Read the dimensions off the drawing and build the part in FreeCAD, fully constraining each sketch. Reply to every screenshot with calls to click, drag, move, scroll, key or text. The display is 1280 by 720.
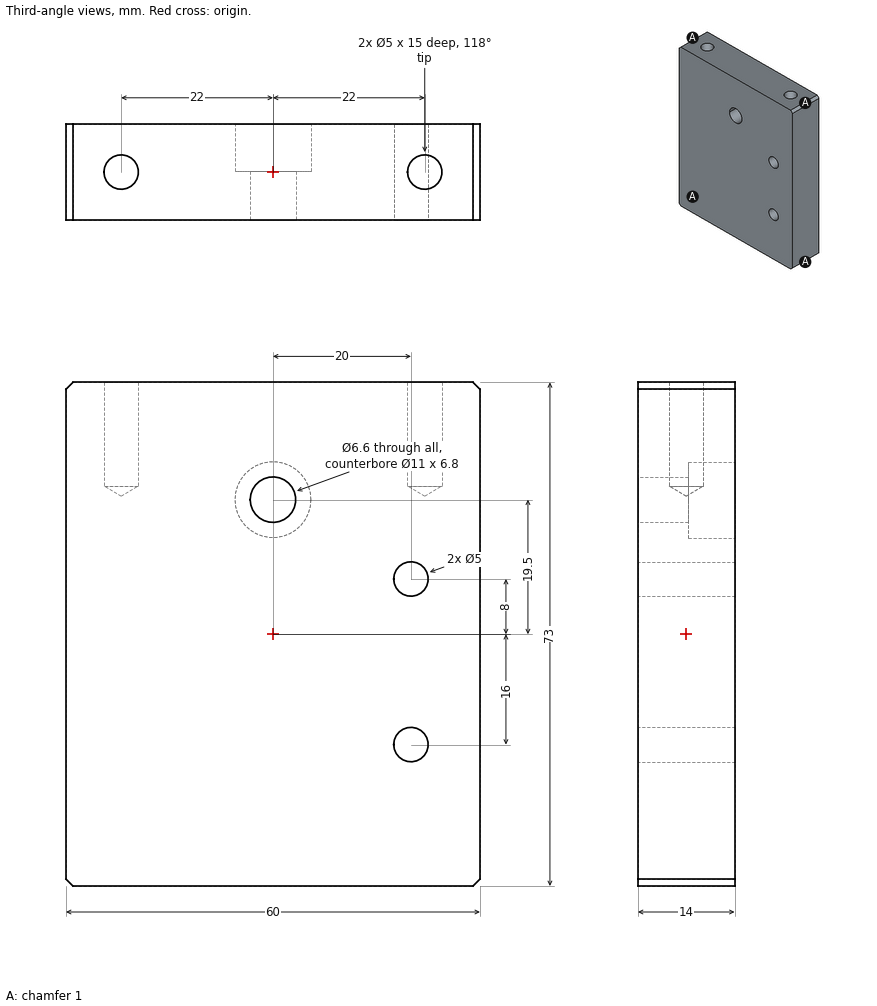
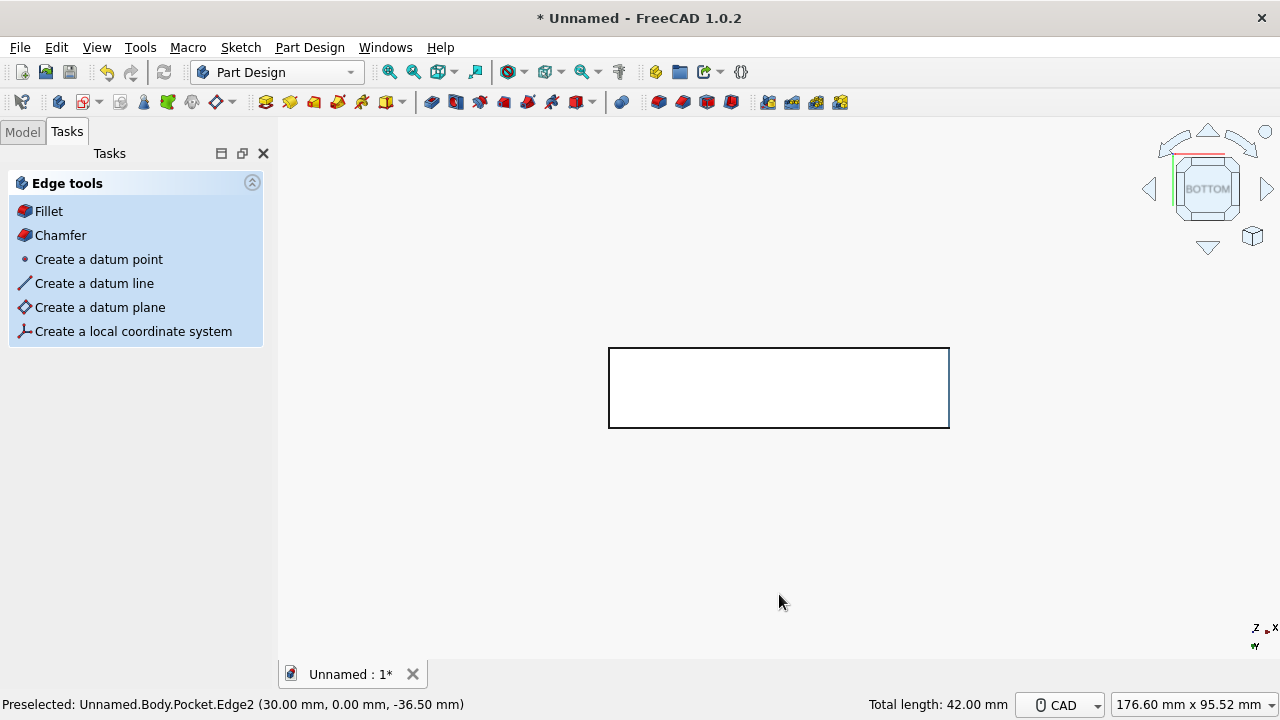
click(390, 72)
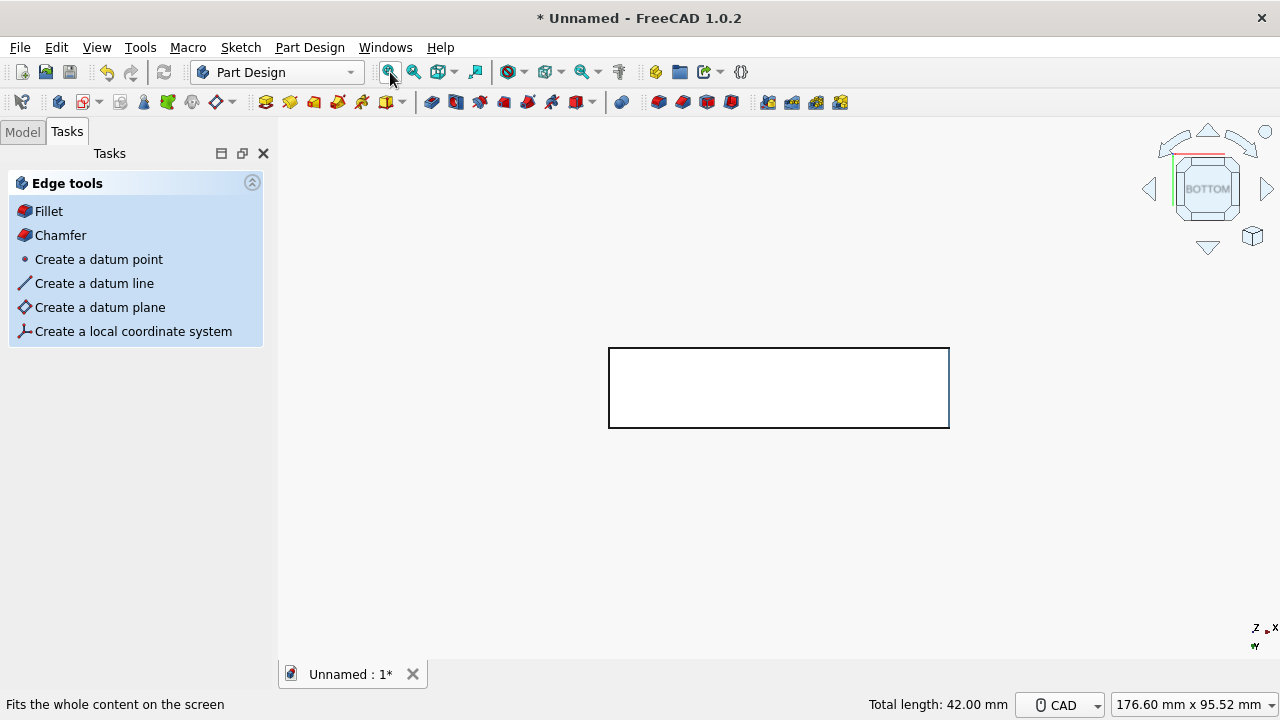
click(609, 387, ctrl)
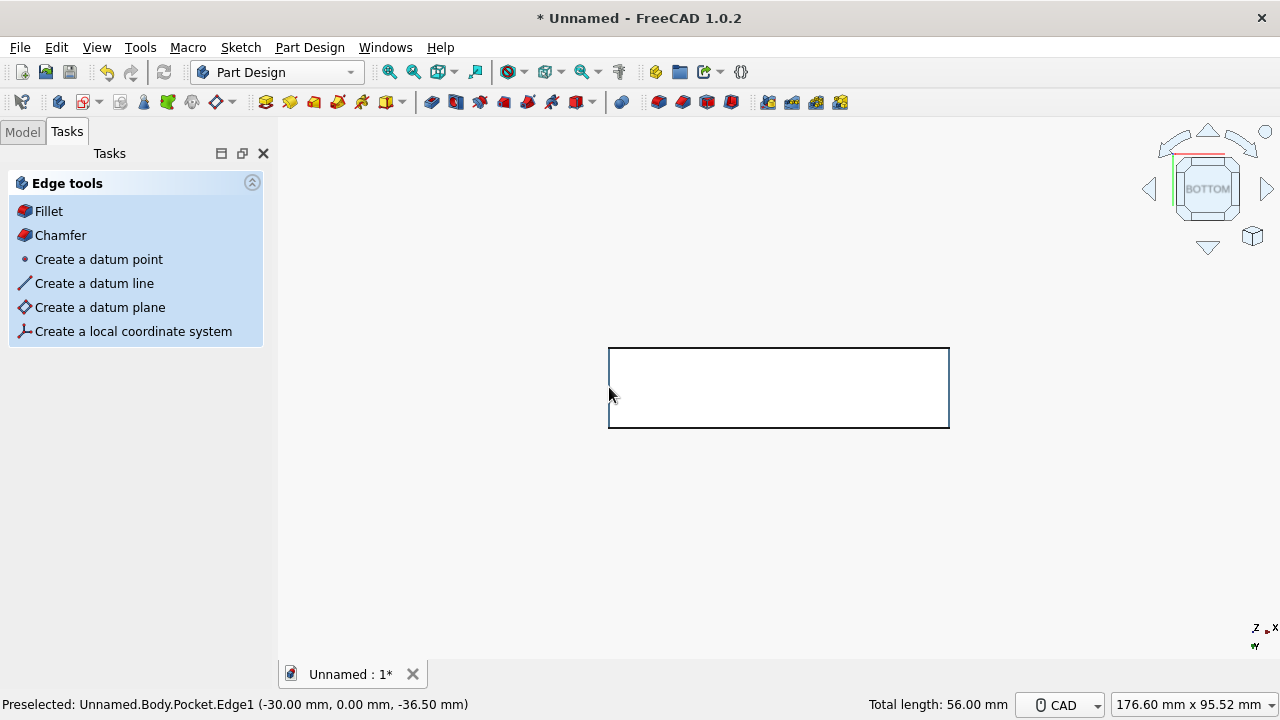
click(684, 102)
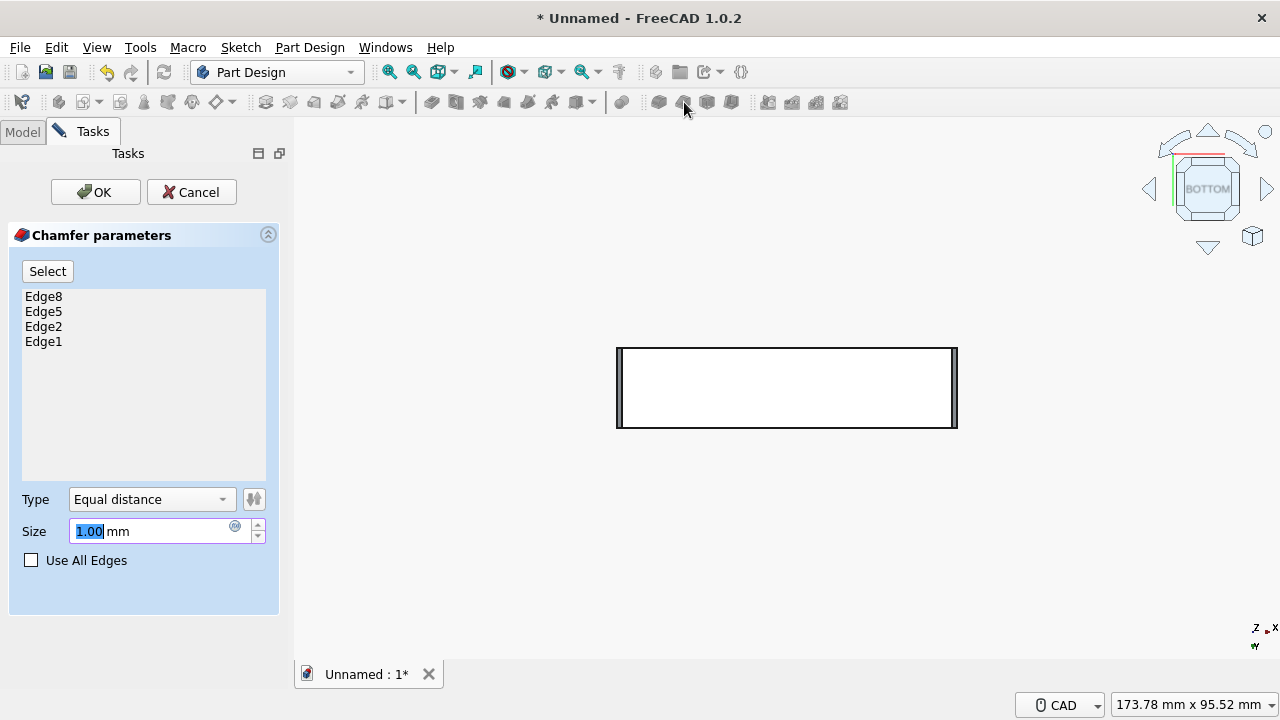
text(1)
key(Tab)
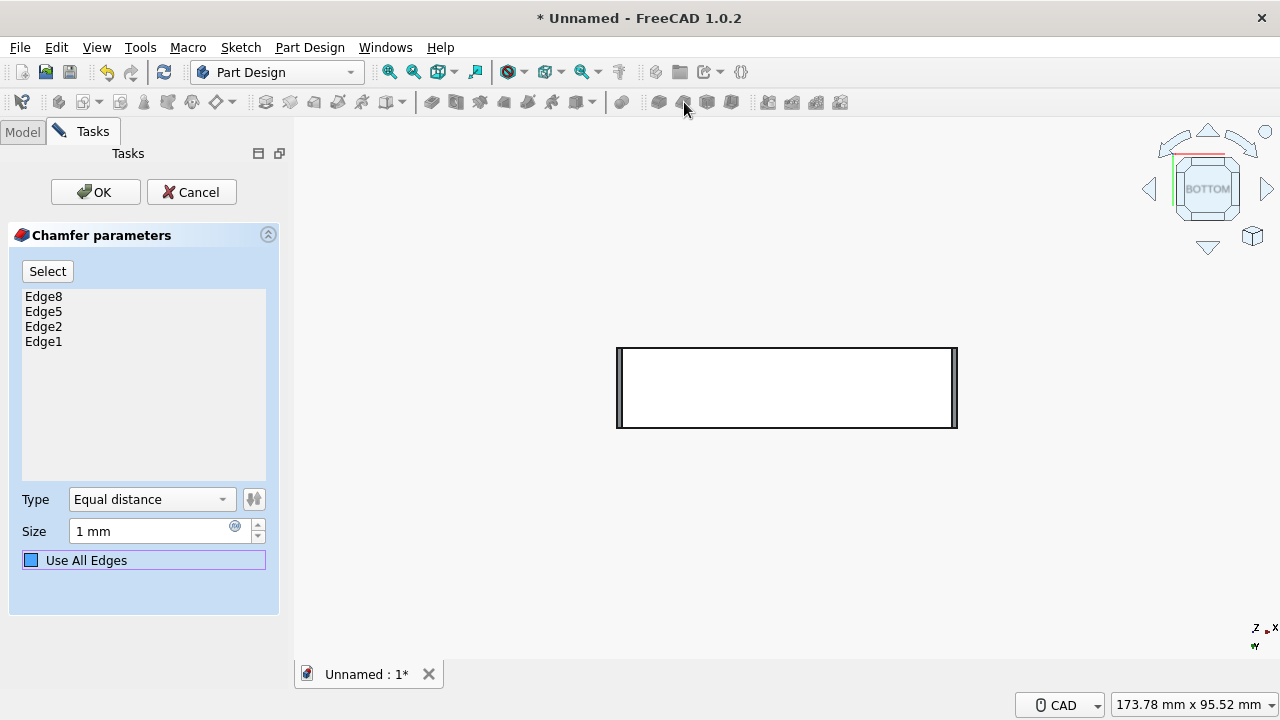
click(96, 192)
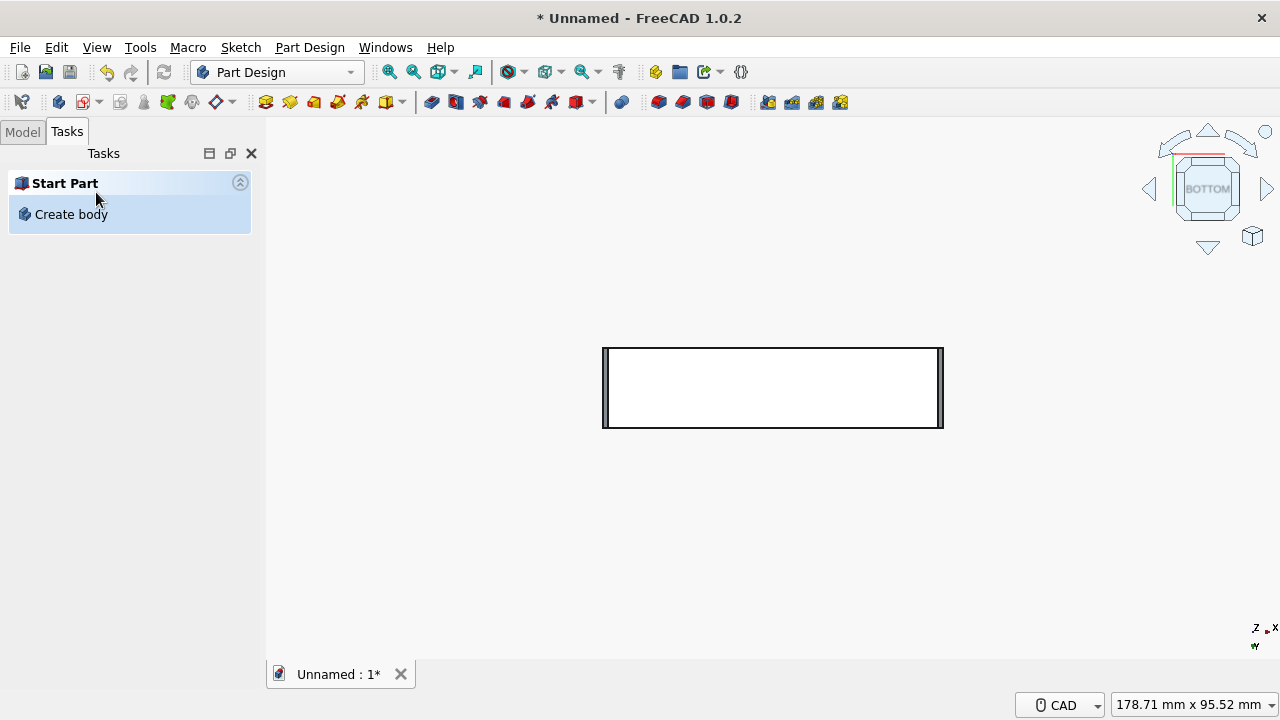
click(390, 72)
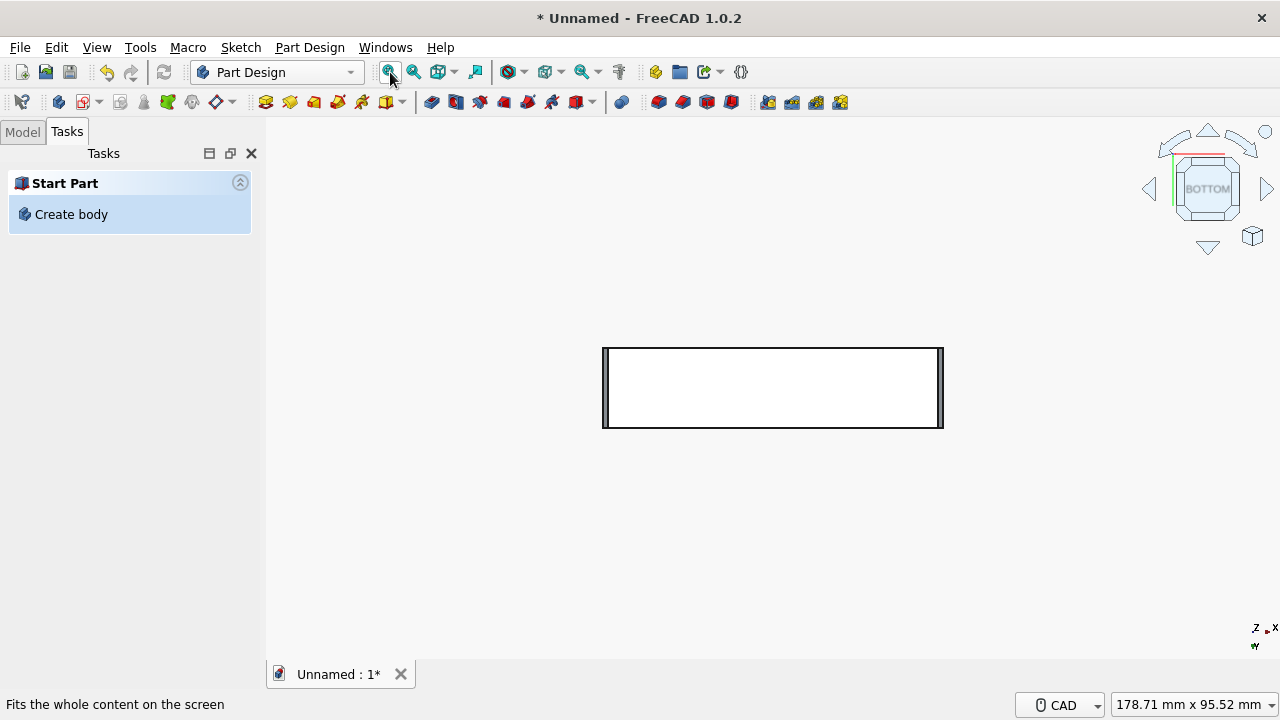
key(4)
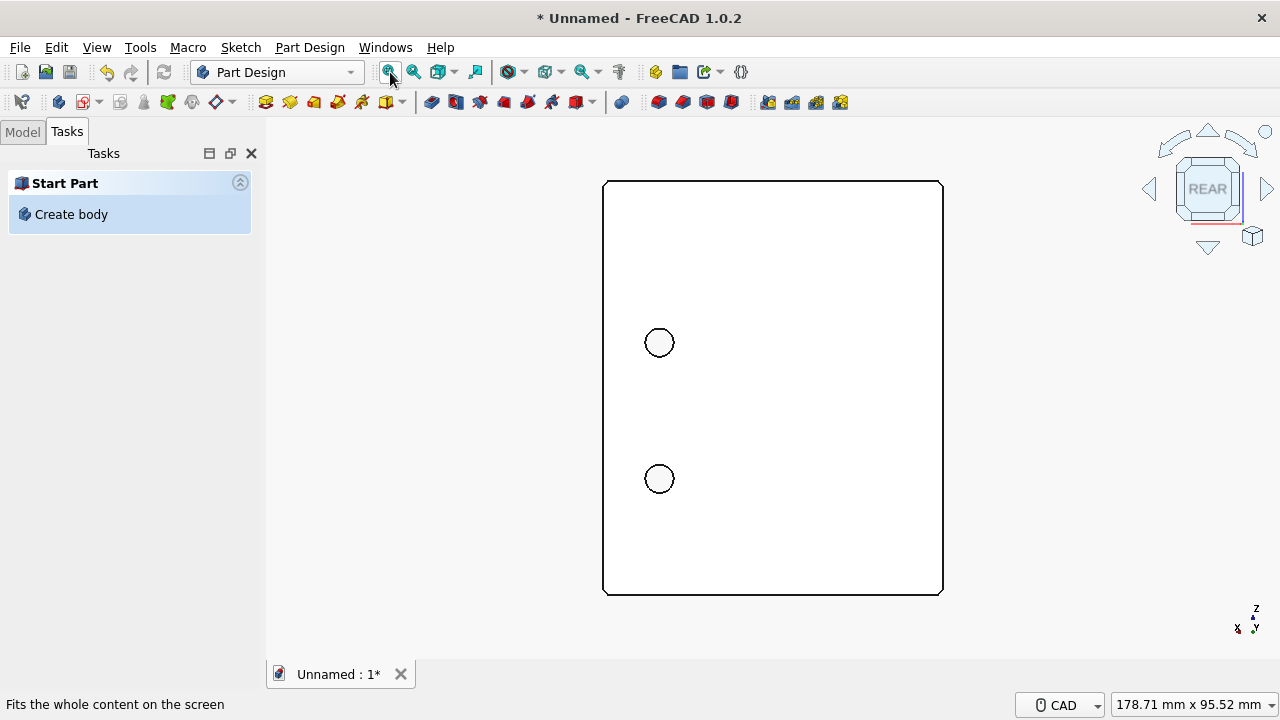
click(822, 328)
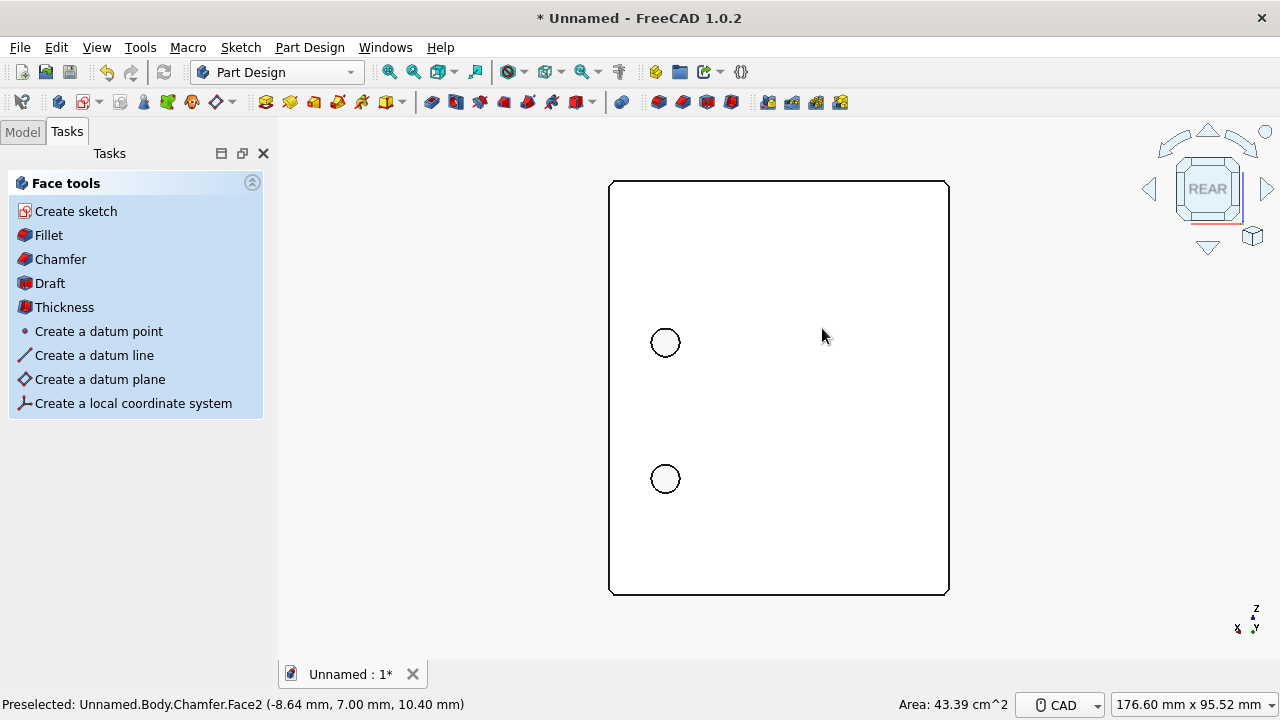
click(84, 102)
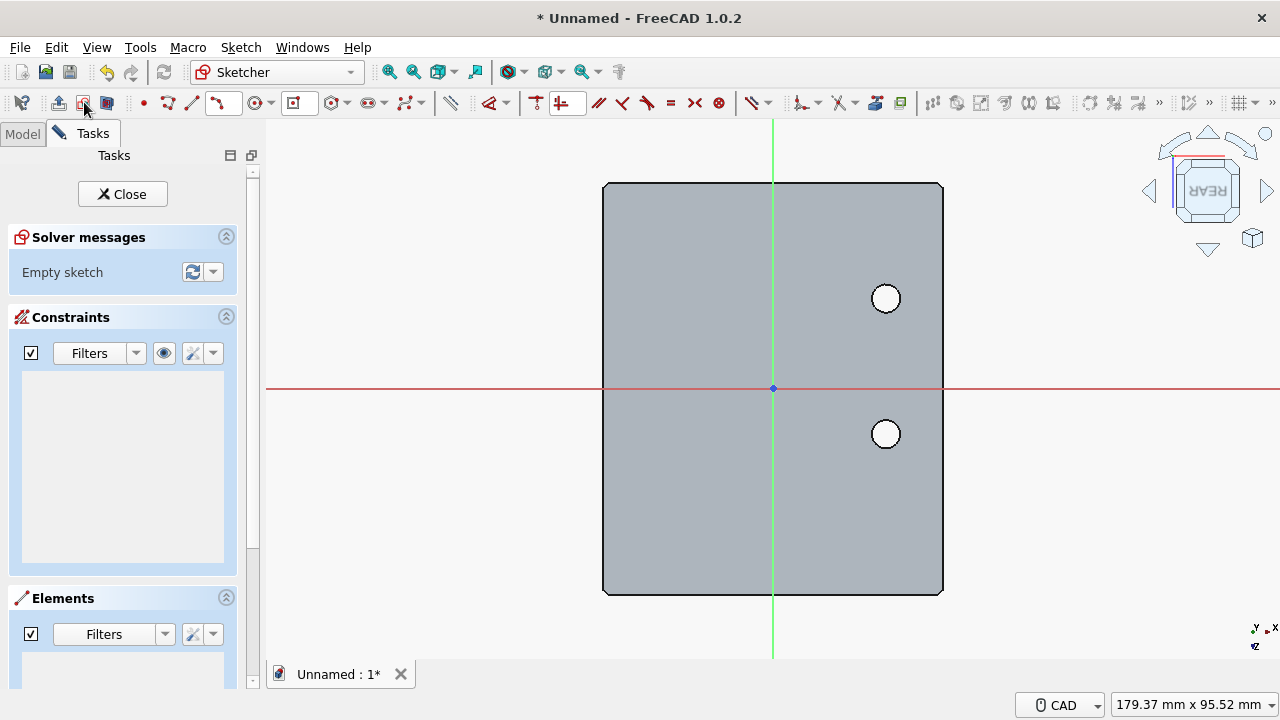
scroll(782, 513, up, 11)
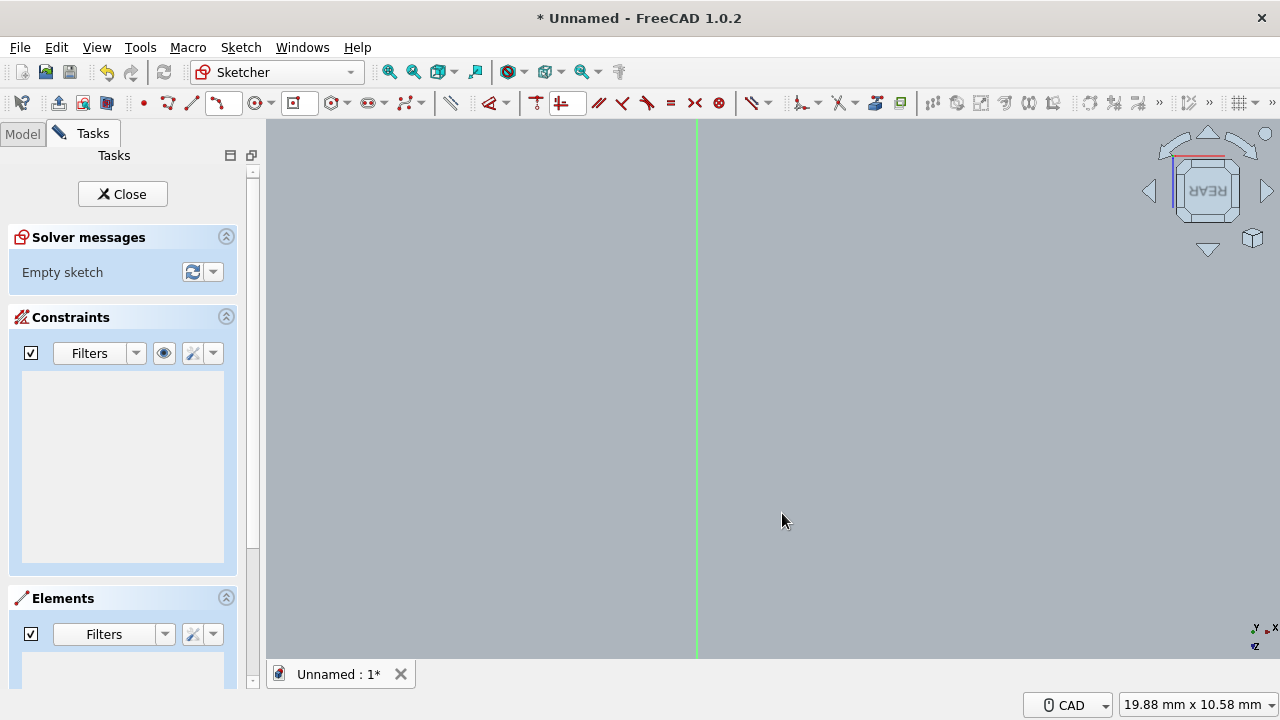
click(256, 104)